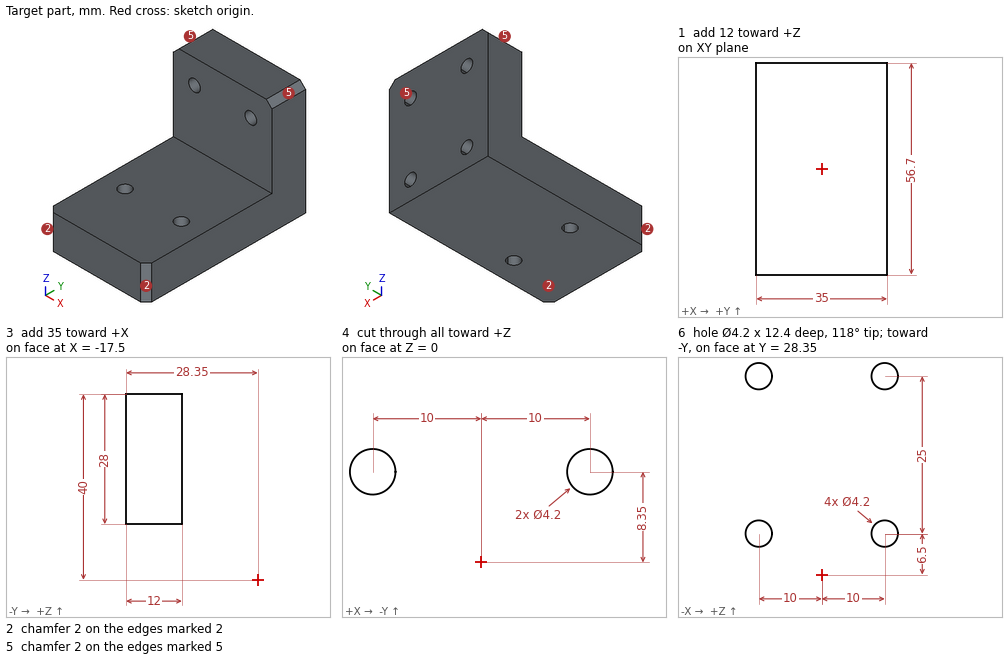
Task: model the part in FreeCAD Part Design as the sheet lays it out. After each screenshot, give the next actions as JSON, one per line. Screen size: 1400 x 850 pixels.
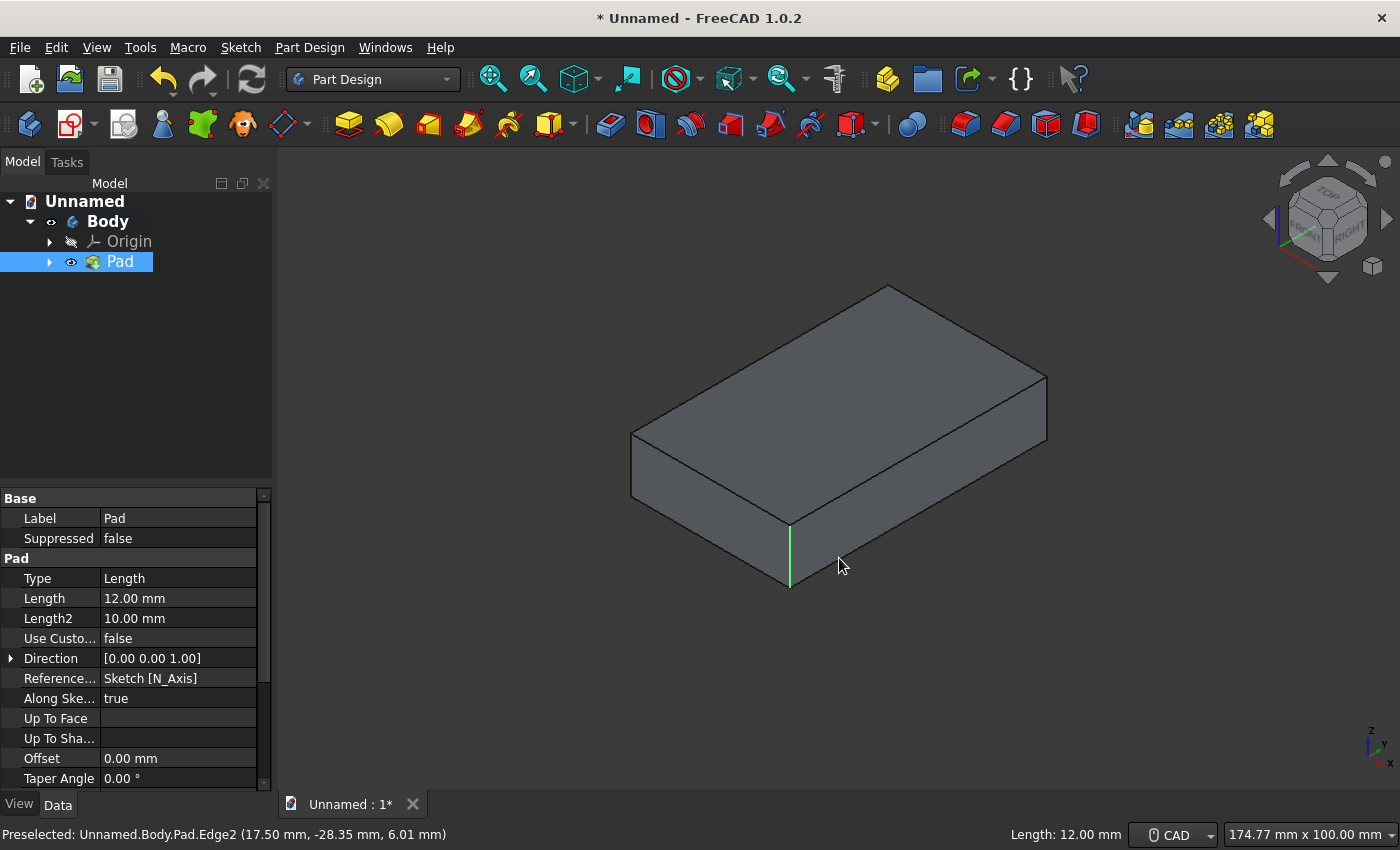
{"action": "key", "text": "2"}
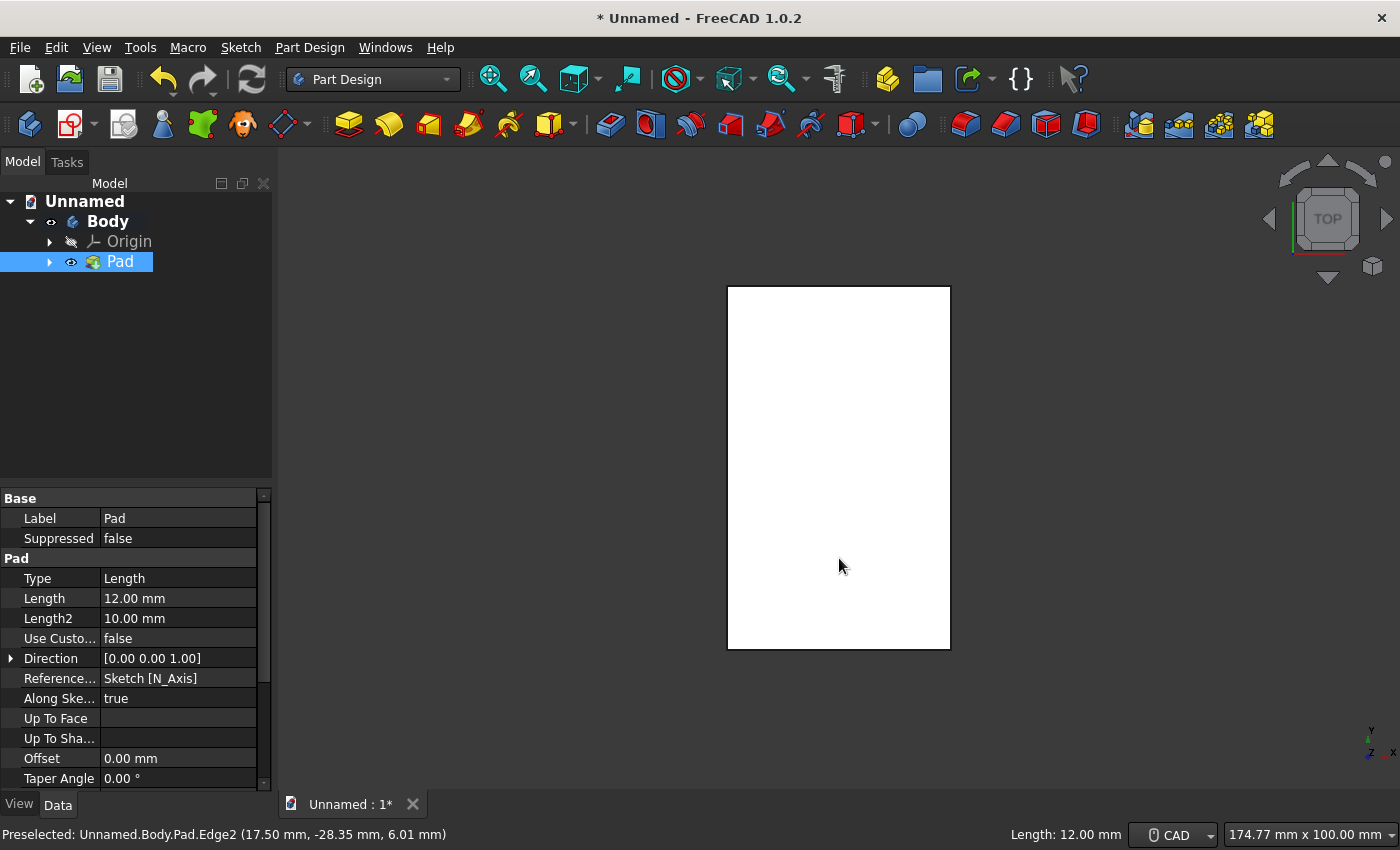
{"action": "key", "text": "1"}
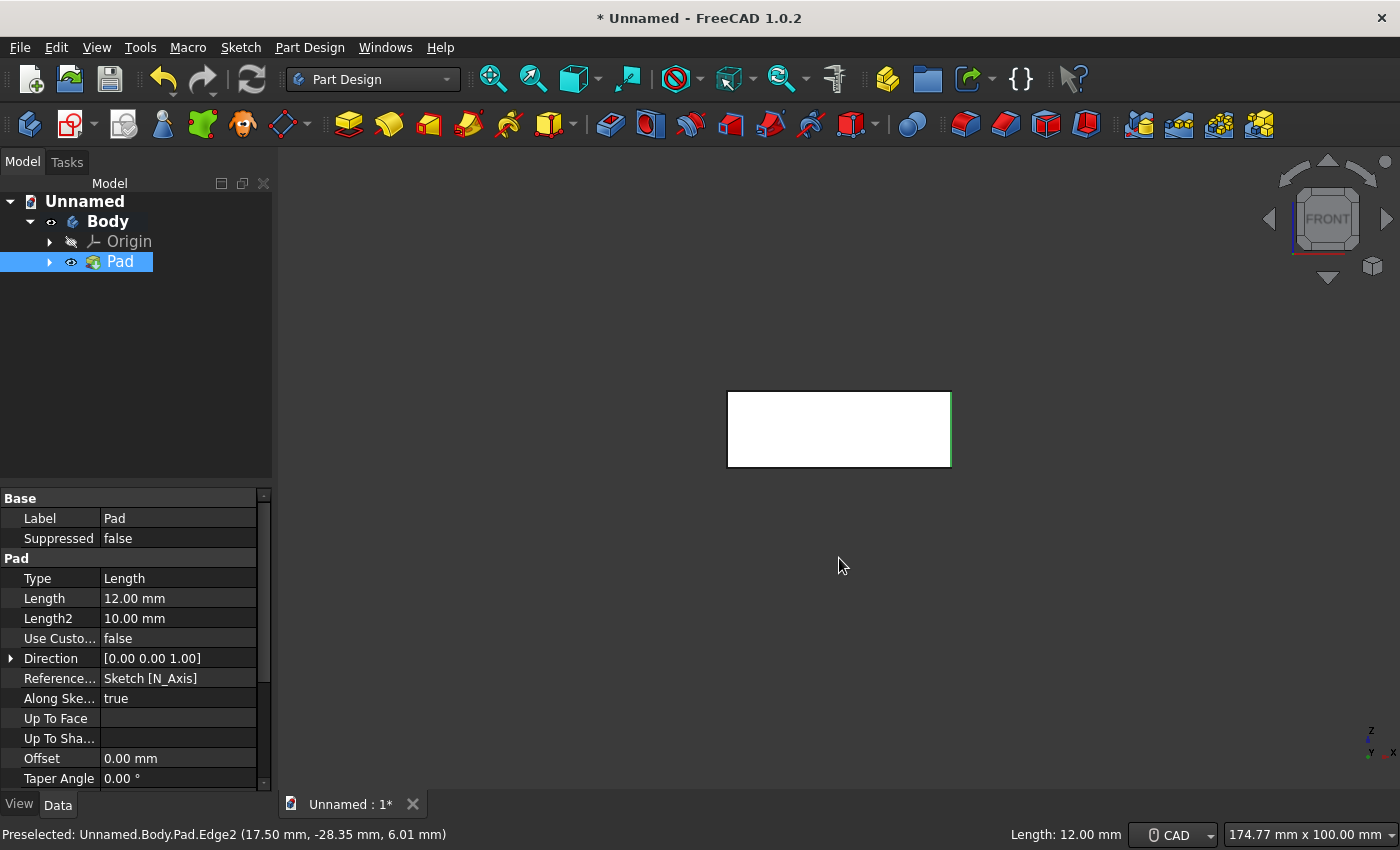
{"action": "left_click", "coordinate": [494, 80]}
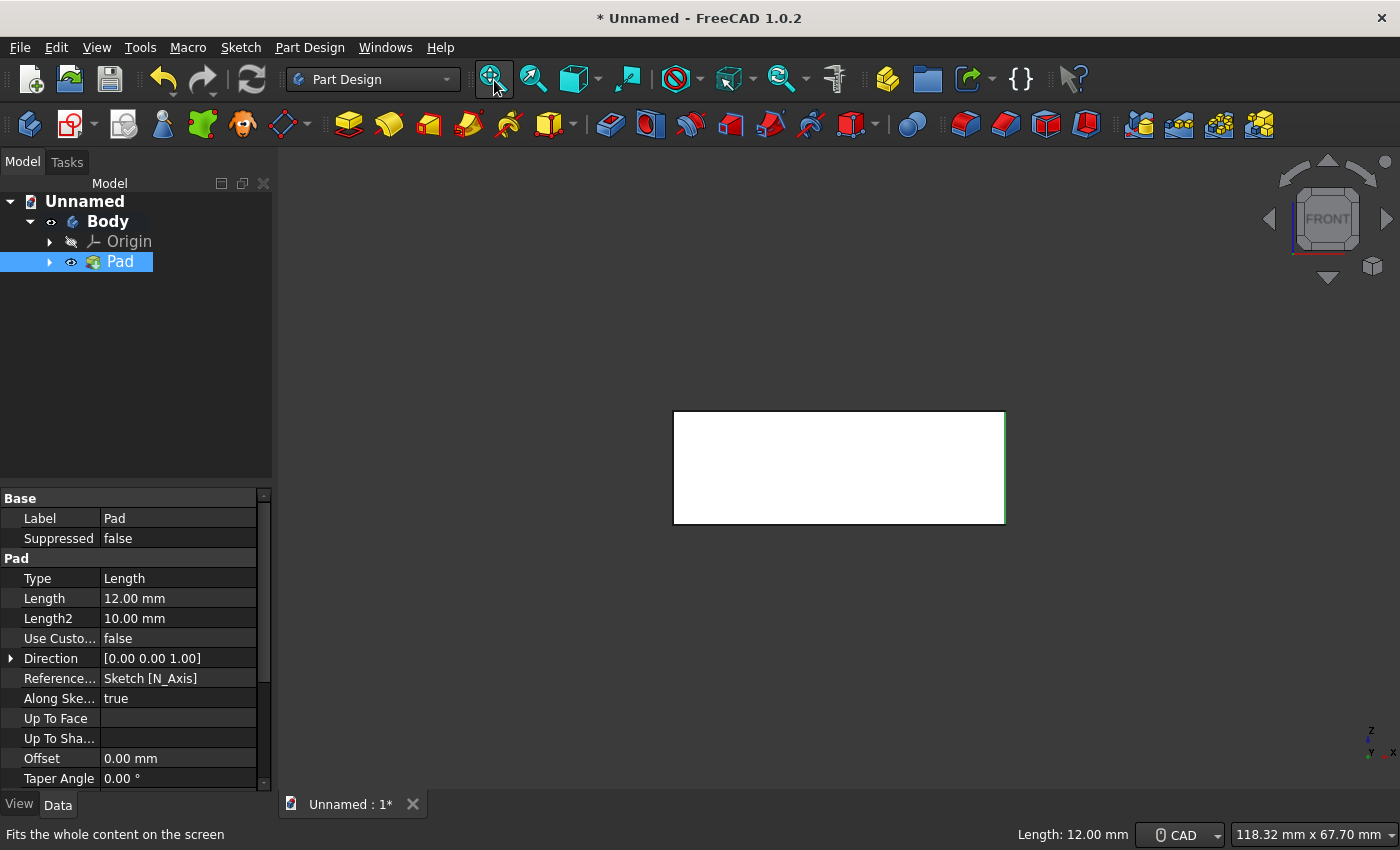
{"action": "left_click", "coordinate": [673, 467], "text": "ctrl"}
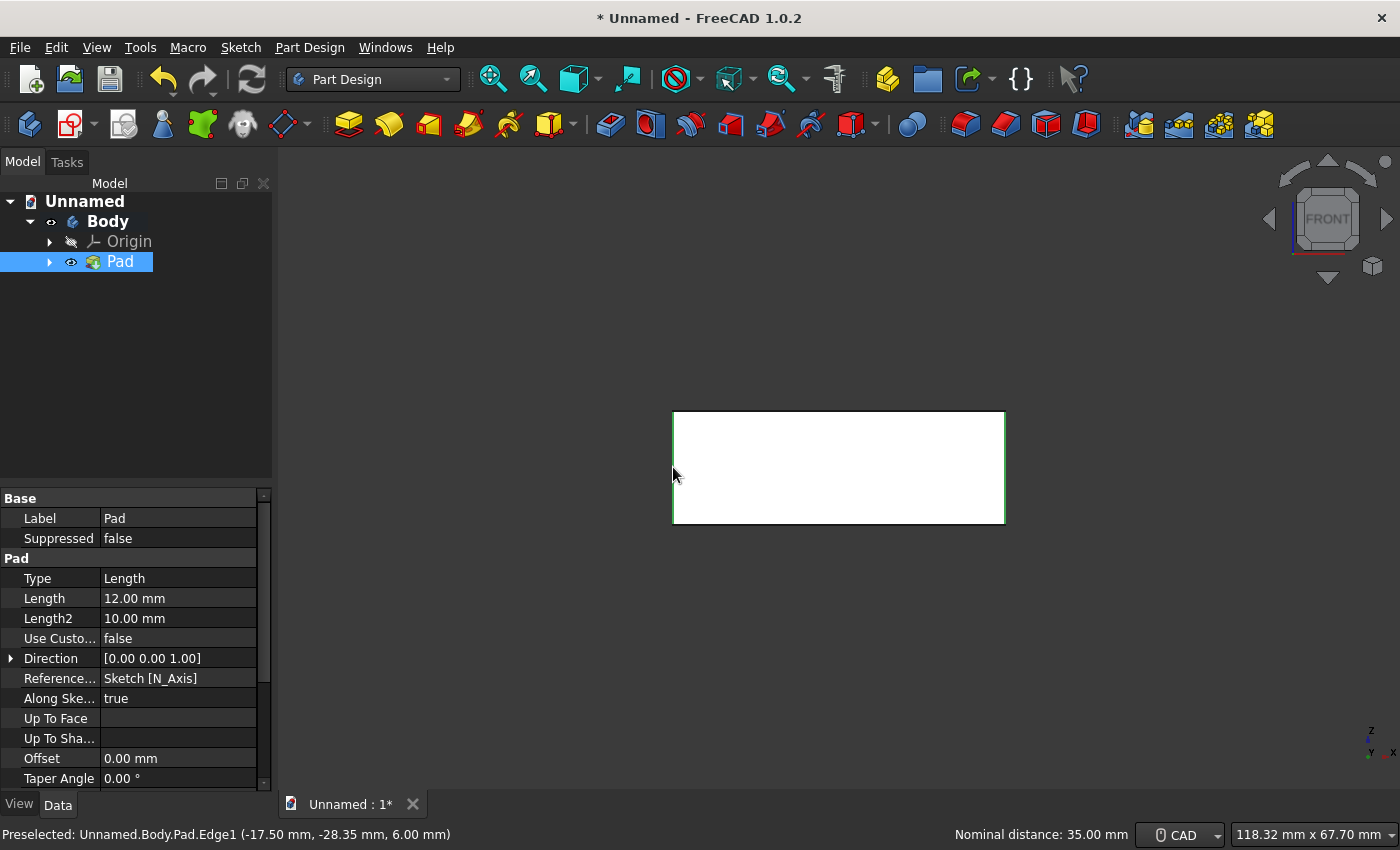
{"action": "left_click", "coordinate": [1006, 124]}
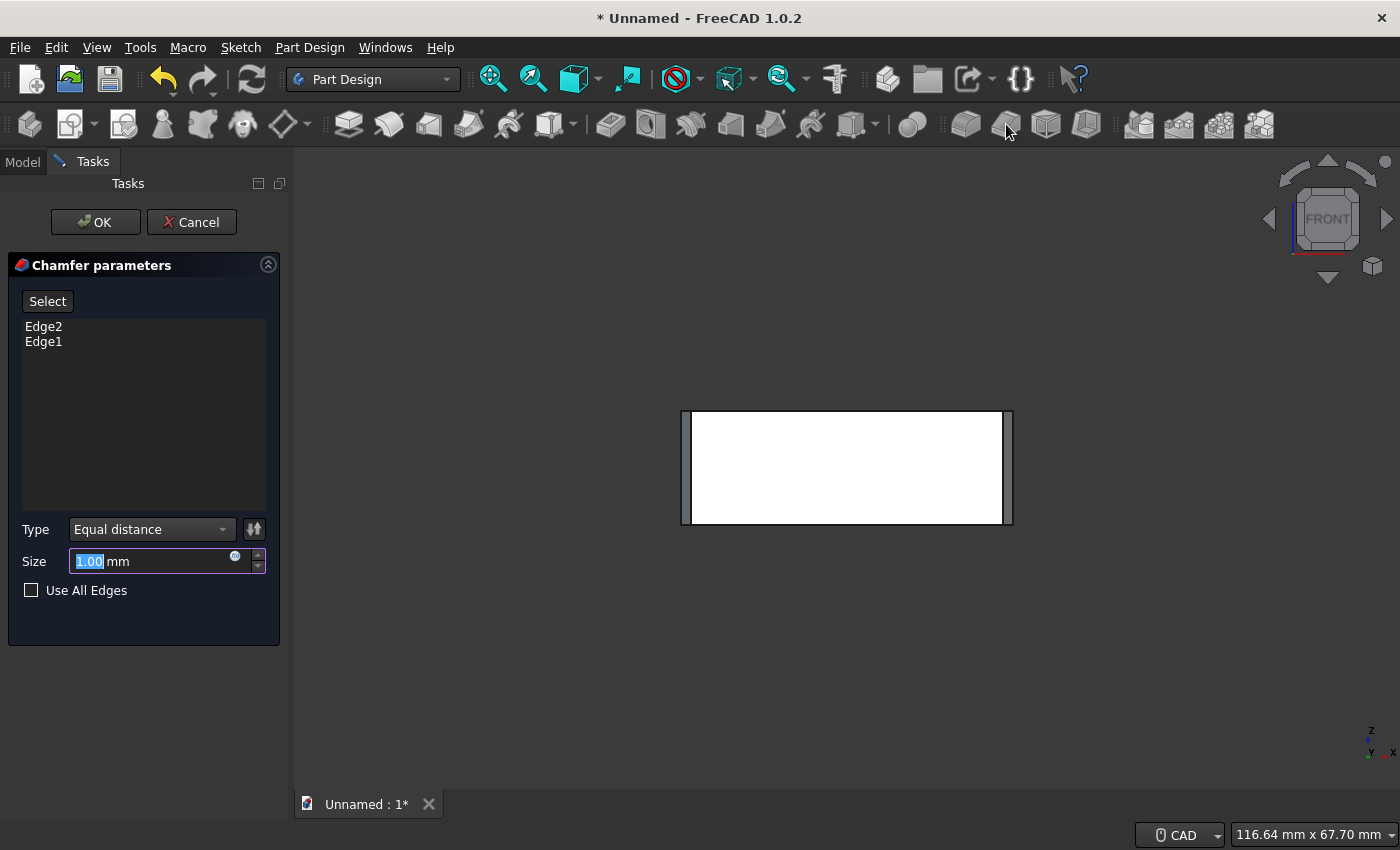
{"action": "type", "text": "2"}
{"action": "key", "text": "Tab"}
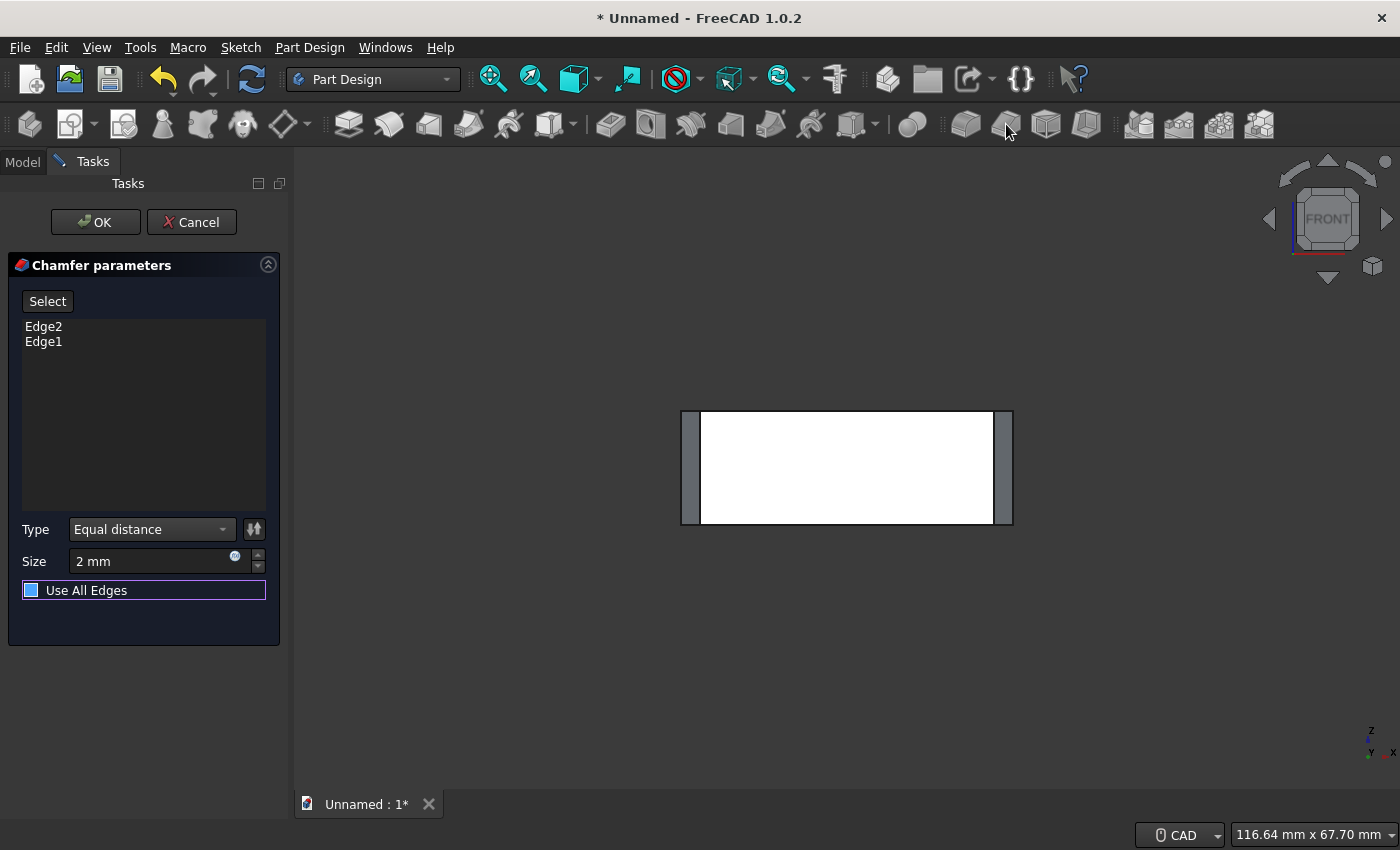
{"action": "left_click", "coordinate": [96, 222]}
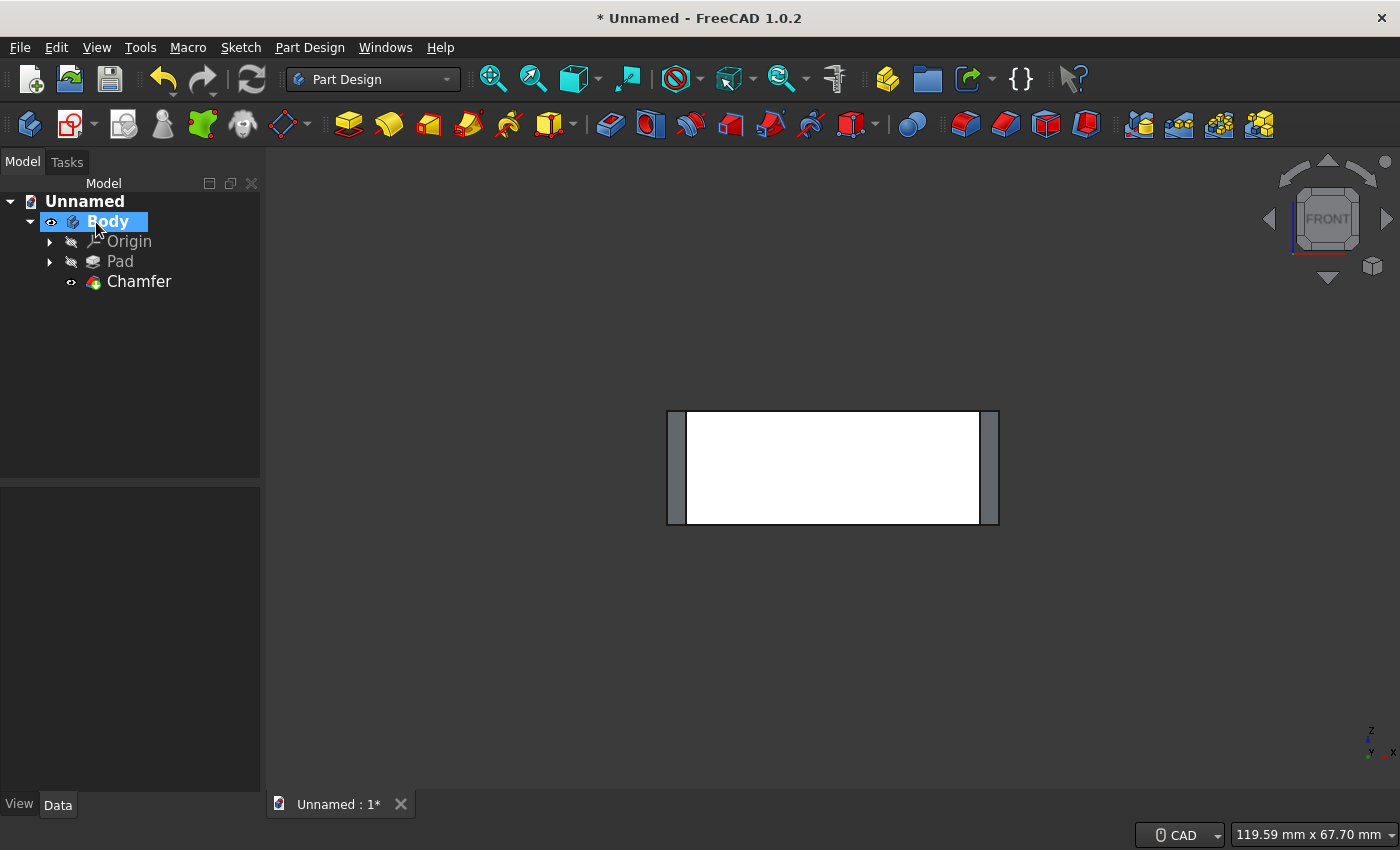
{"action": "left_click", "coordinate": [494, 80]}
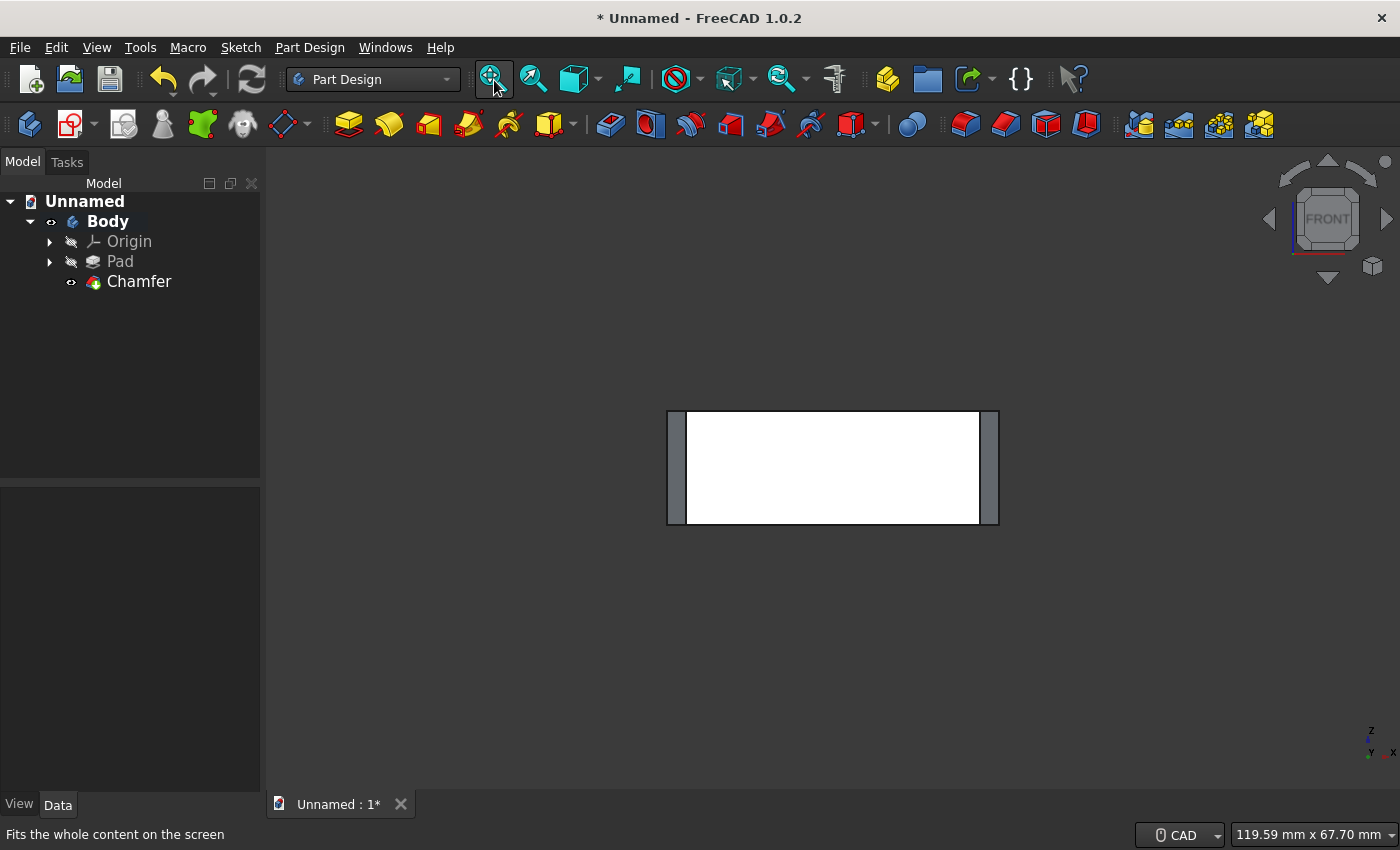
{"action": "key", "text": "6"}